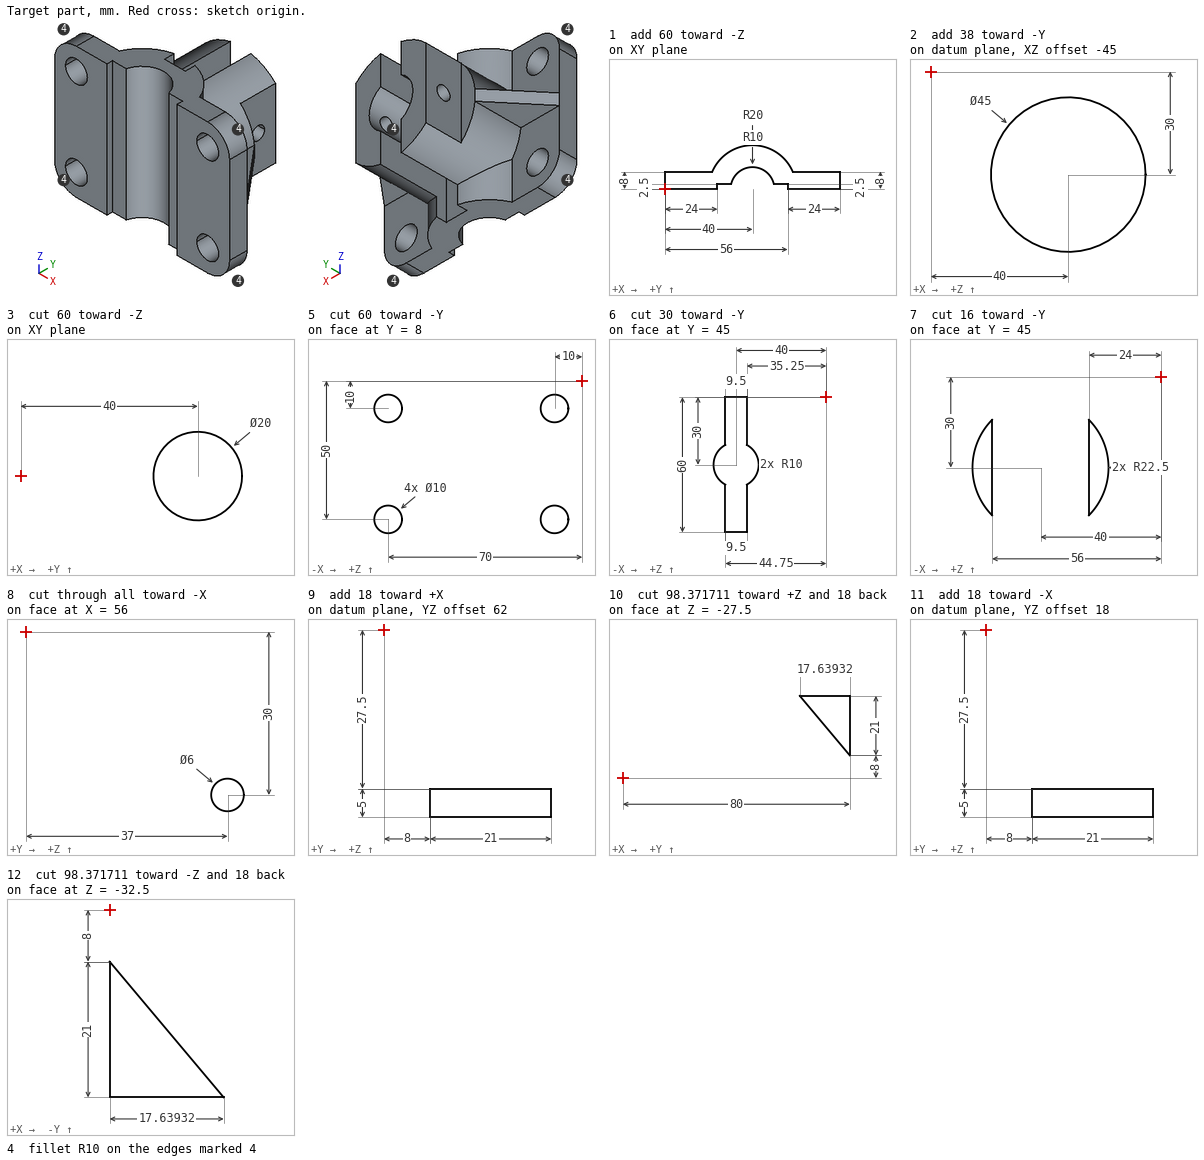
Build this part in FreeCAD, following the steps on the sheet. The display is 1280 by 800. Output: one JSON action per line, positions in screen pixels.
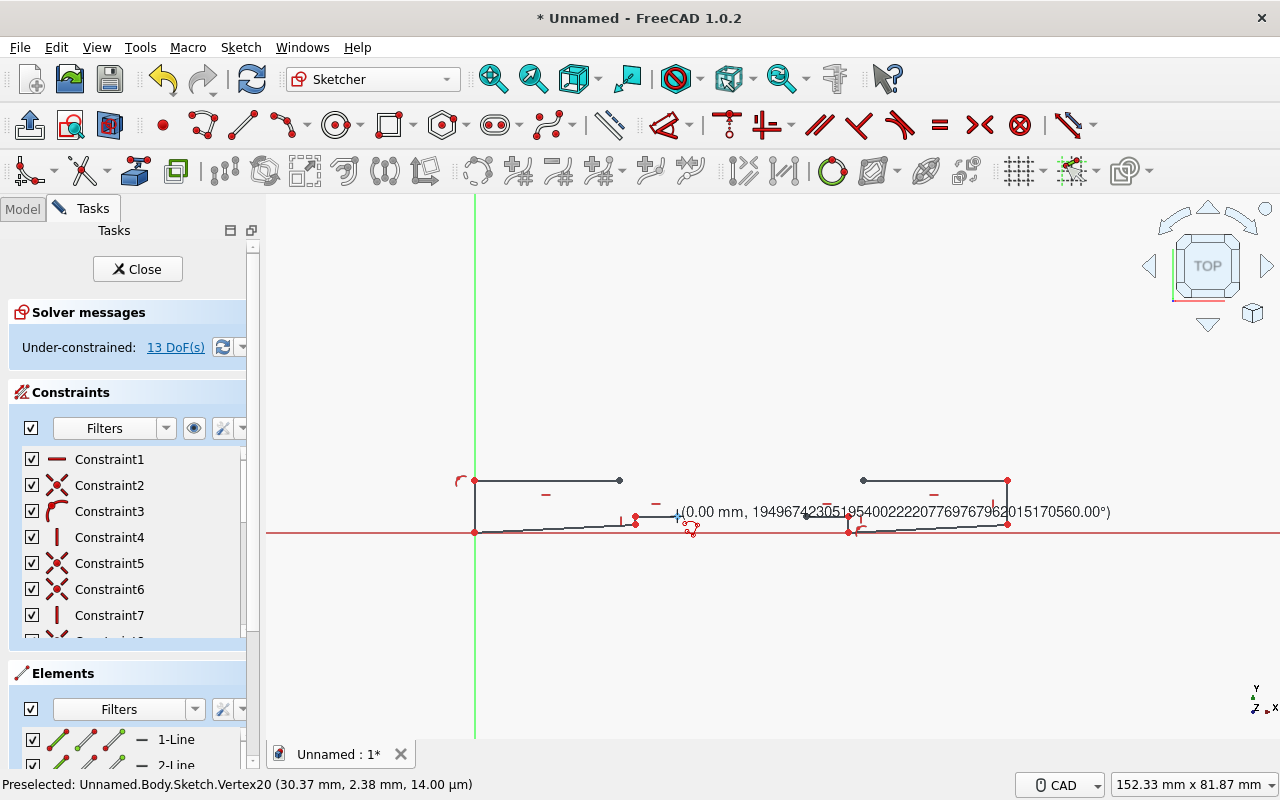
{"action": "left_click", "coordinate": [284, 126]}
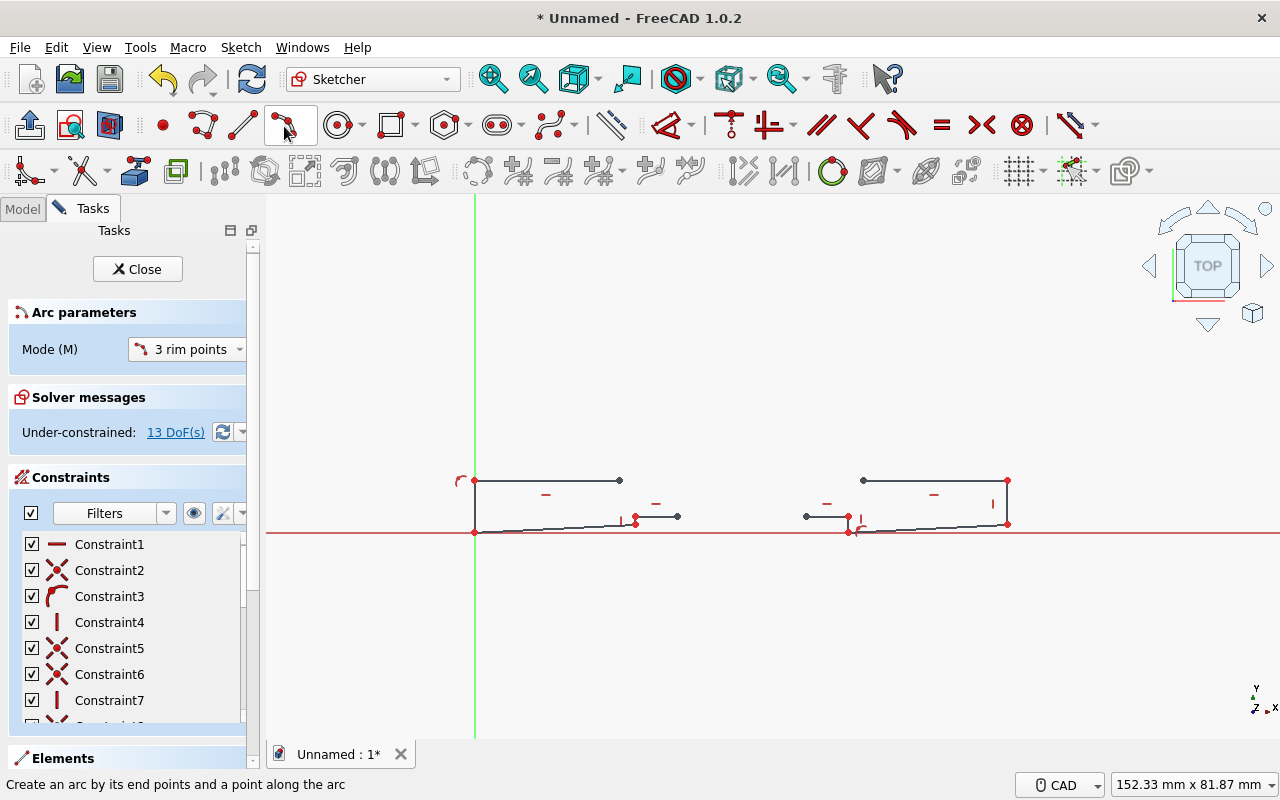
{"action": "left_click", "coordinate": [863, 481]}
{"action": "left_click", "coordinate": [619, 481]}
{"action": "left_click", "coordinate": [741, 400]}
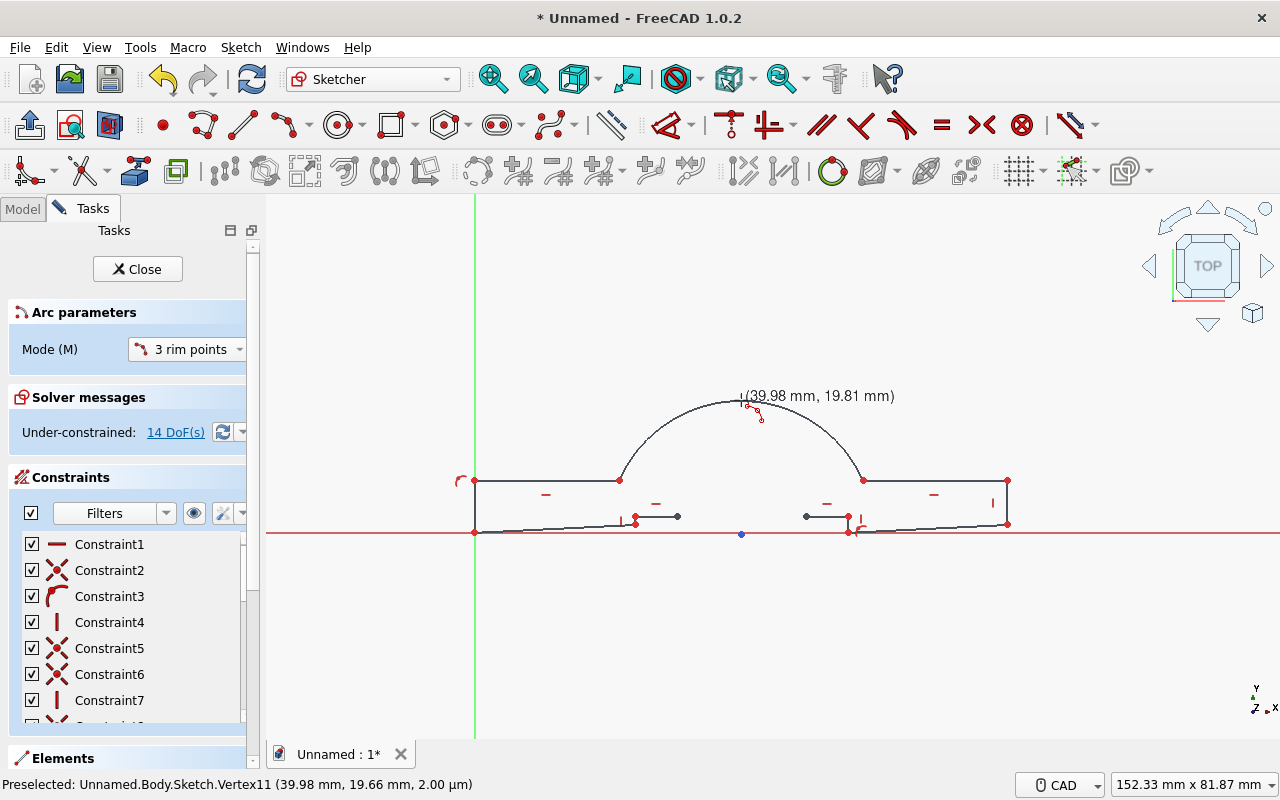
{"action": "left_click", "coordinate": [677, 517]}
{"action": "left_click", "coordinate": [806, 517]}
{"action": "left_click", "coordinate": [741, 466]}
{"action": "key", "text": "Escape"}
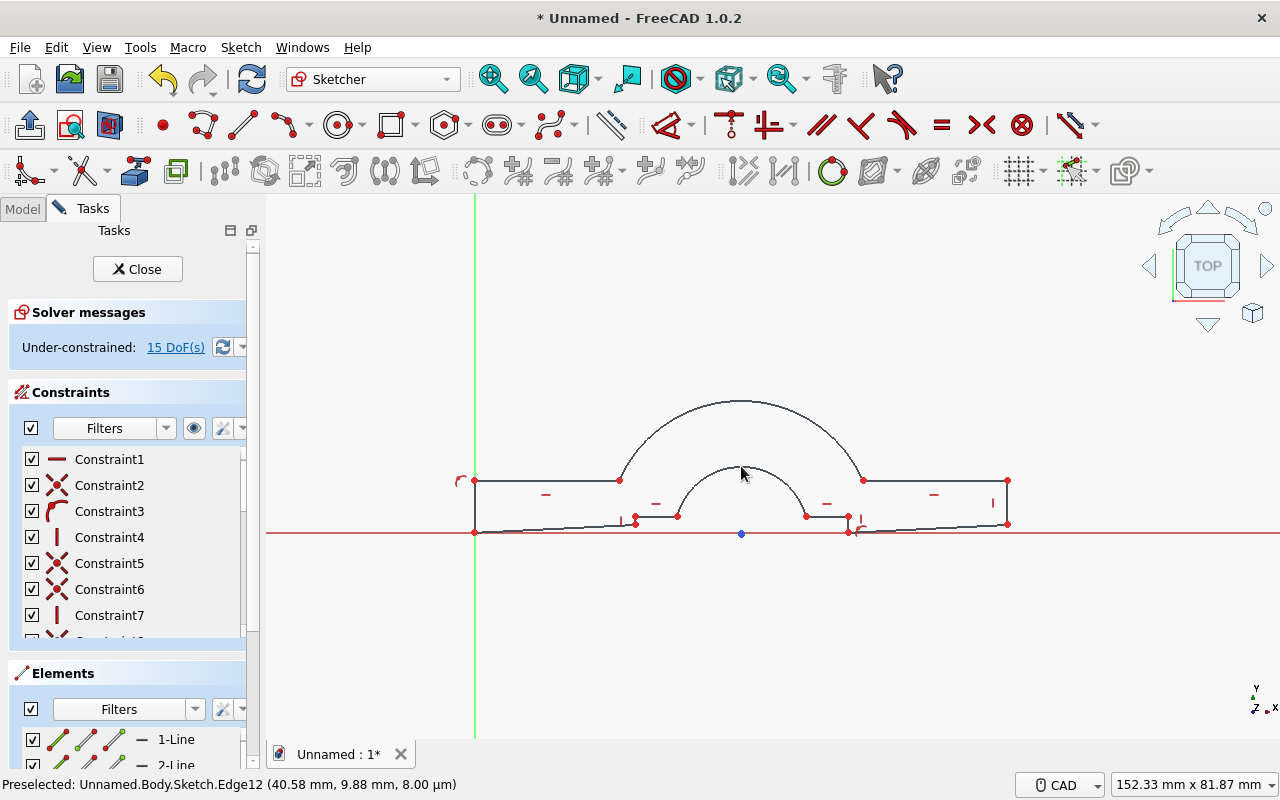
{"action": "left_click", "coordinate": [896, 531]}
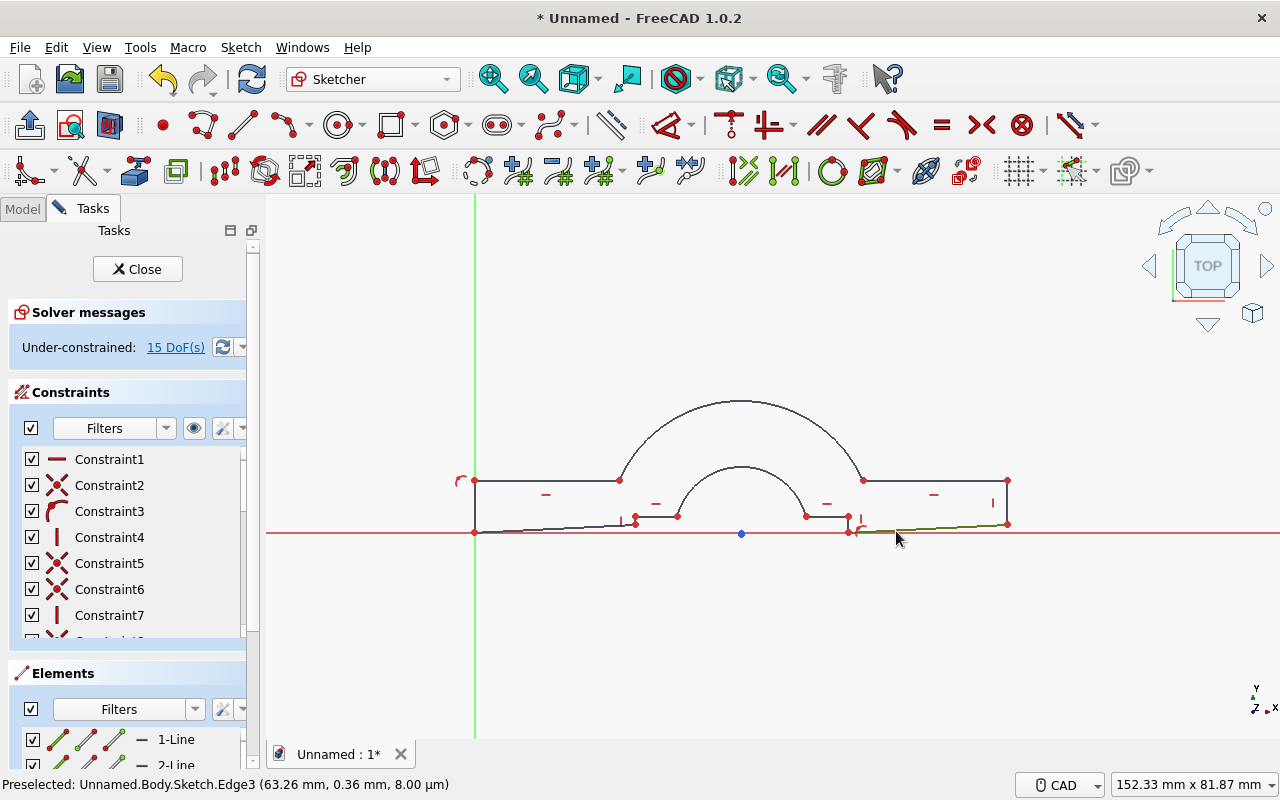
{"action": "key", "text": "h"}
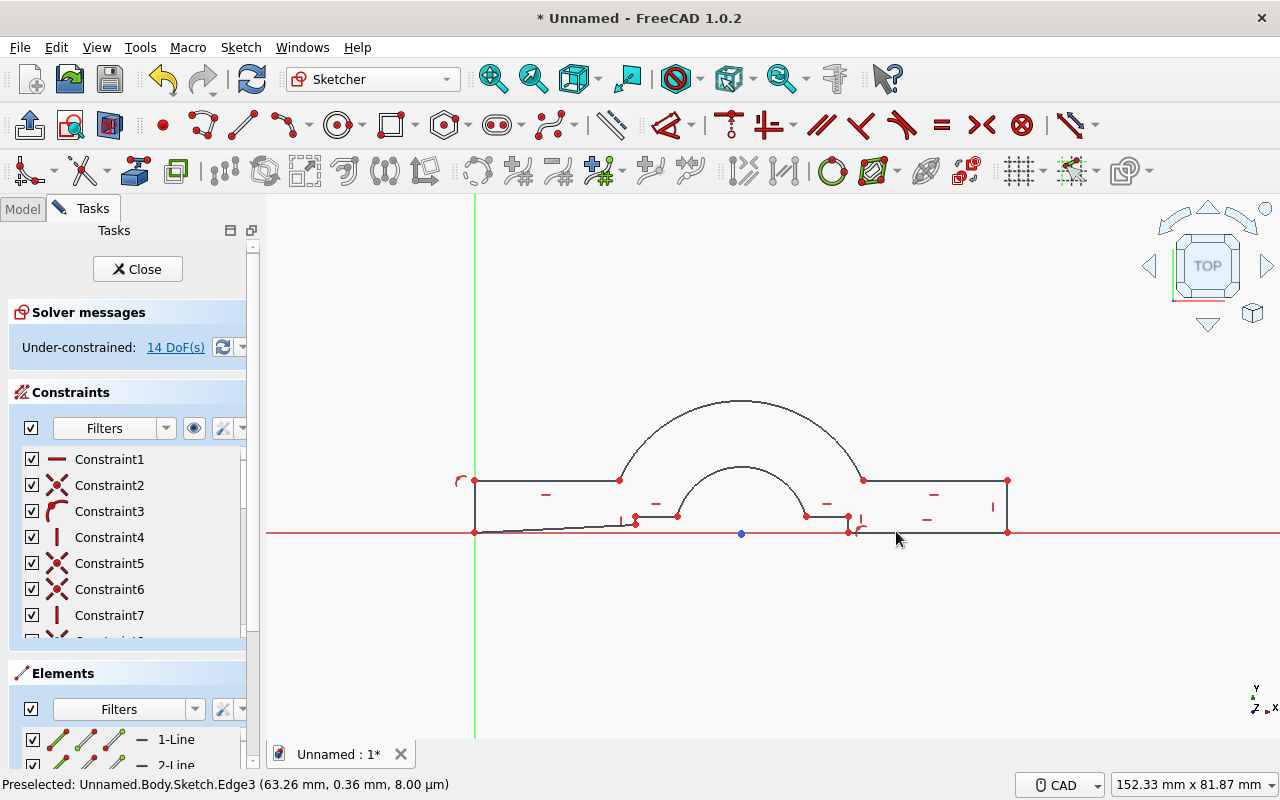
{"action": "left_click", "coordinate": [523, 531]}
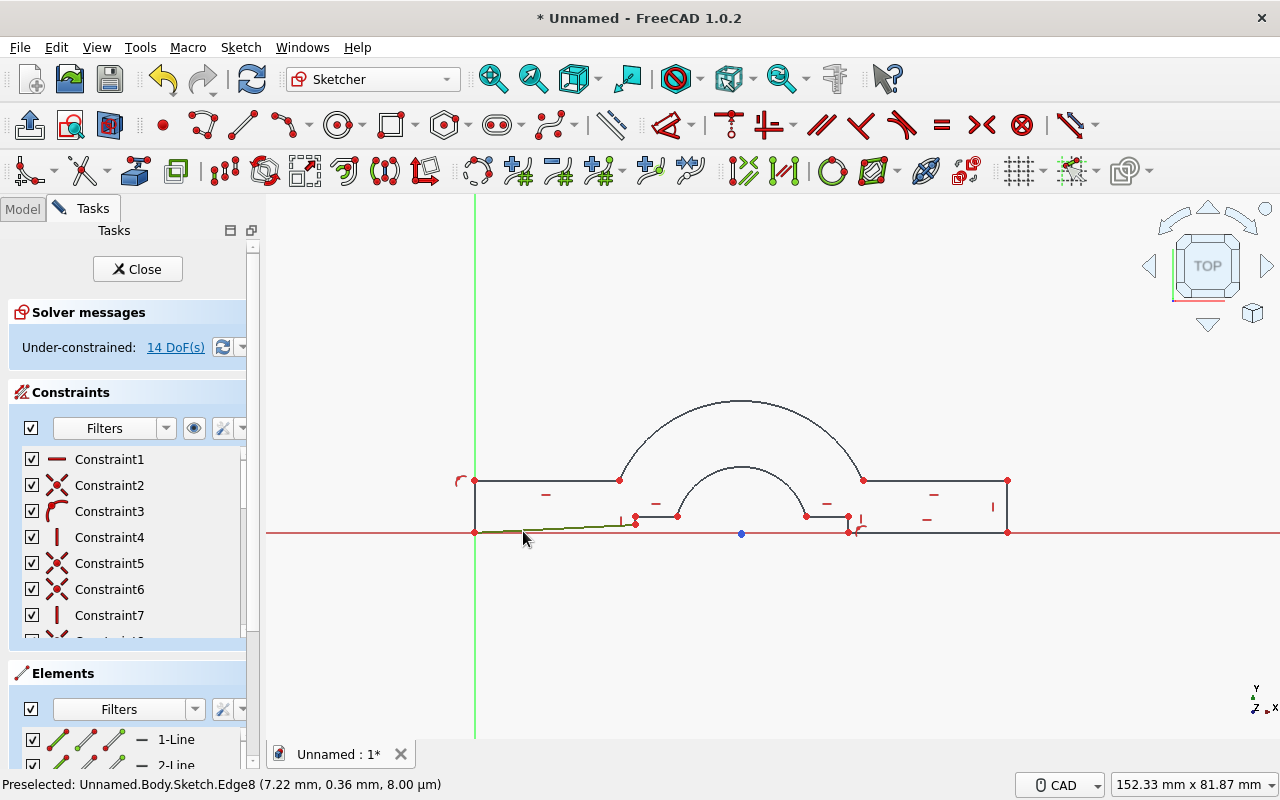
{"action": "key", "text": "h"}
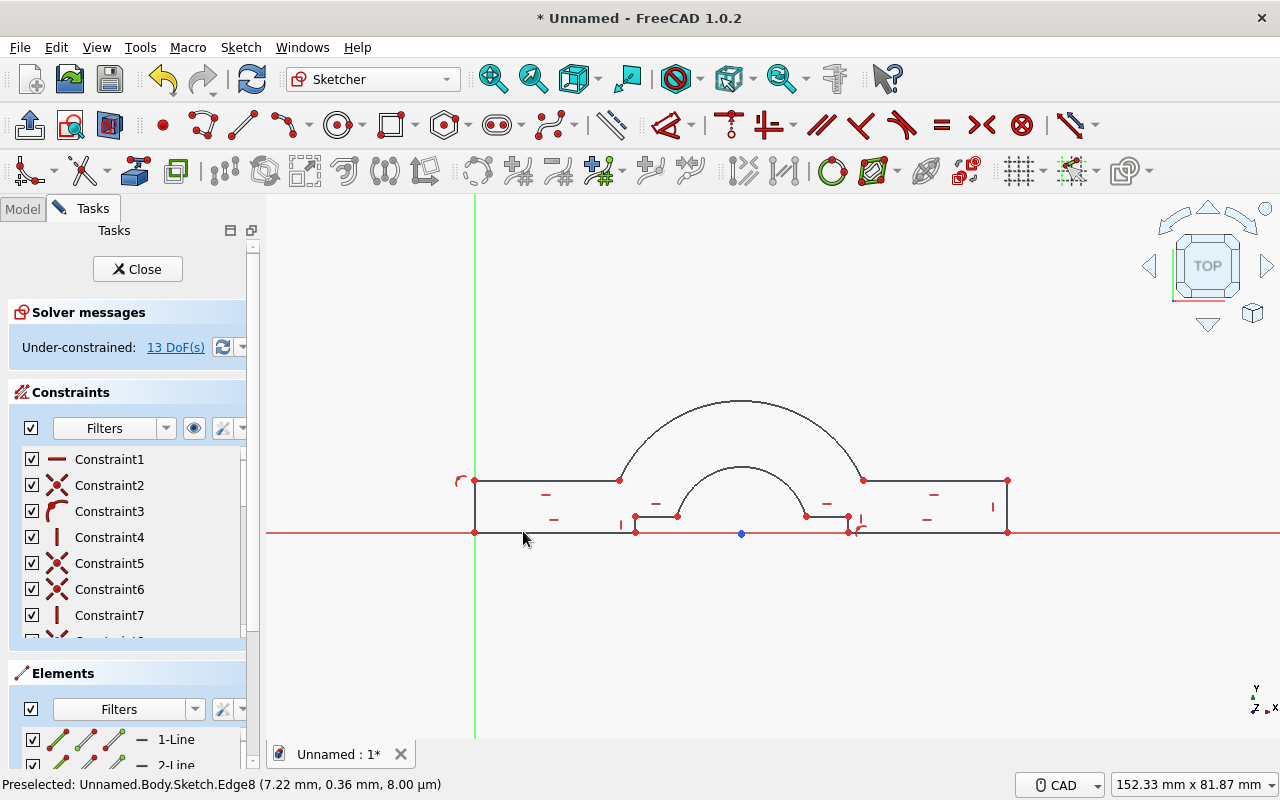
{"action": "left_click", "coordinate": [801, 415]}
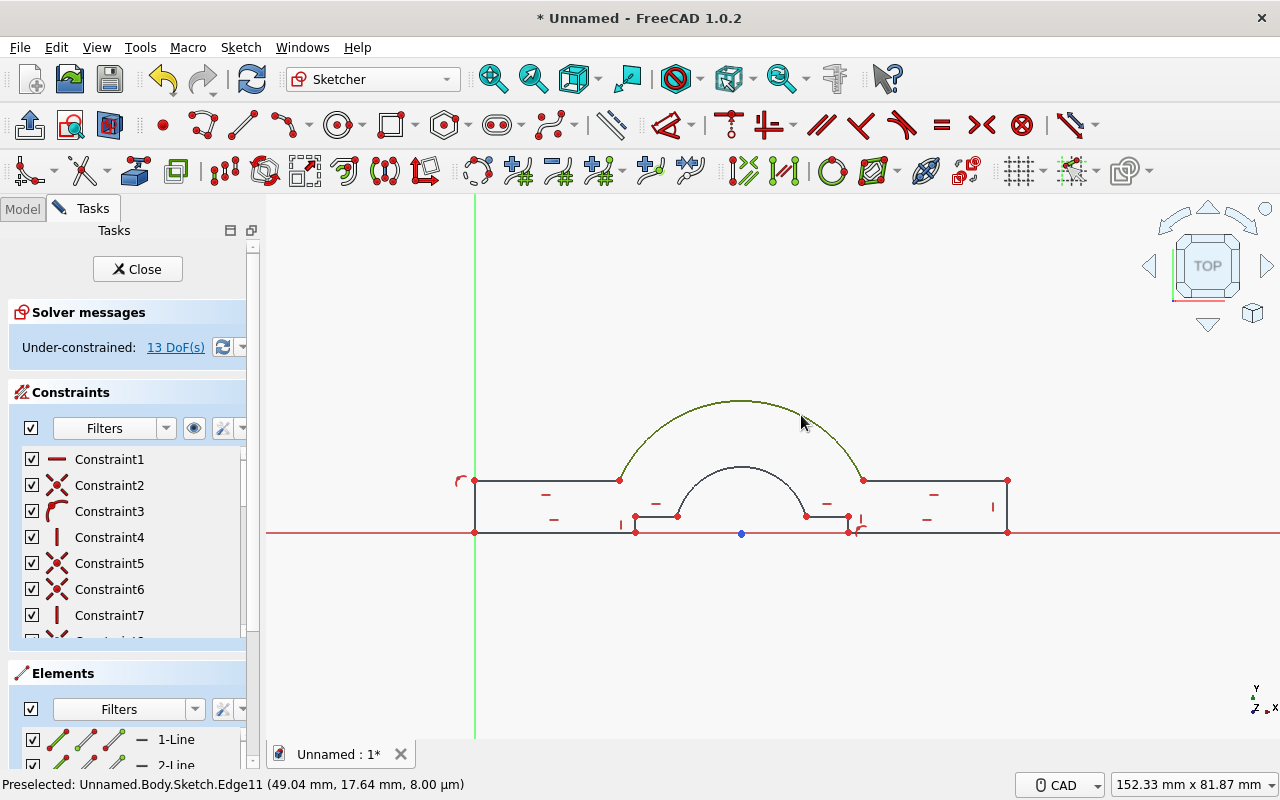
{"action": "left_click", "coordinate": [775, 476]}